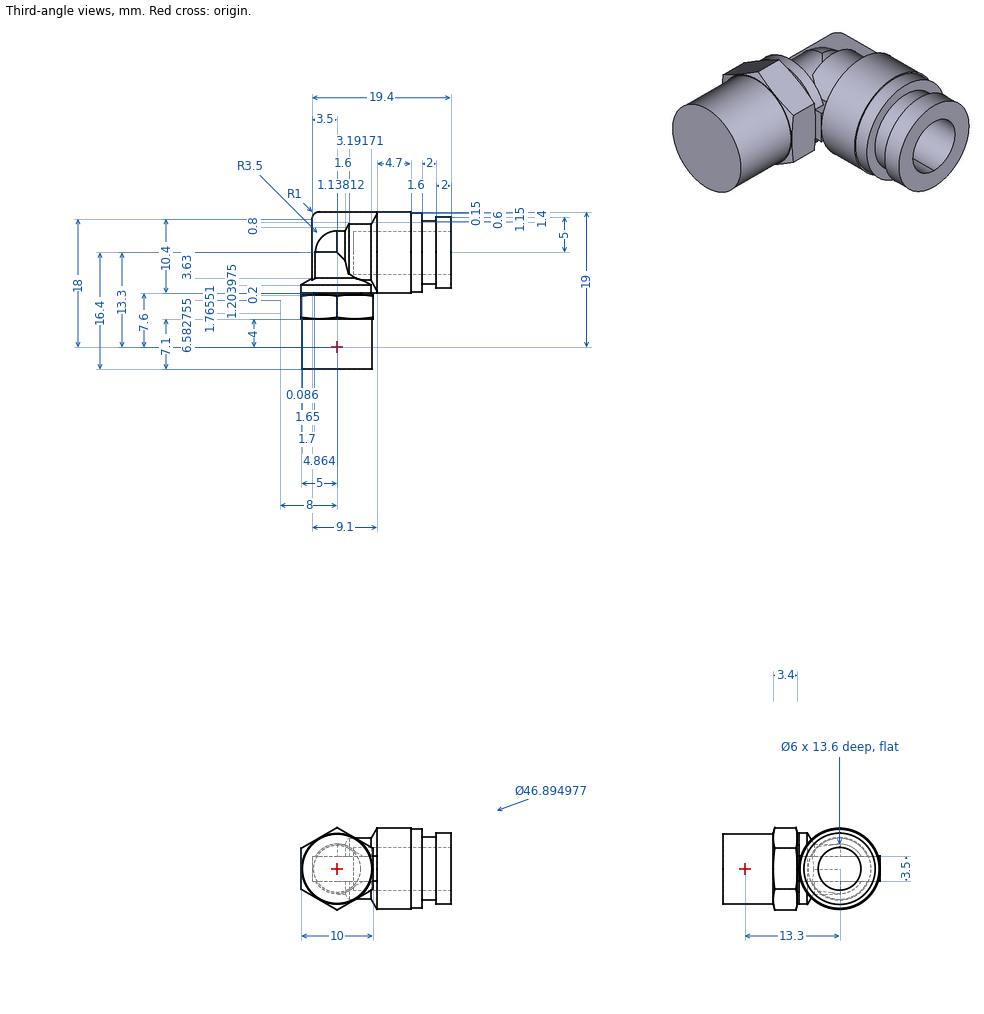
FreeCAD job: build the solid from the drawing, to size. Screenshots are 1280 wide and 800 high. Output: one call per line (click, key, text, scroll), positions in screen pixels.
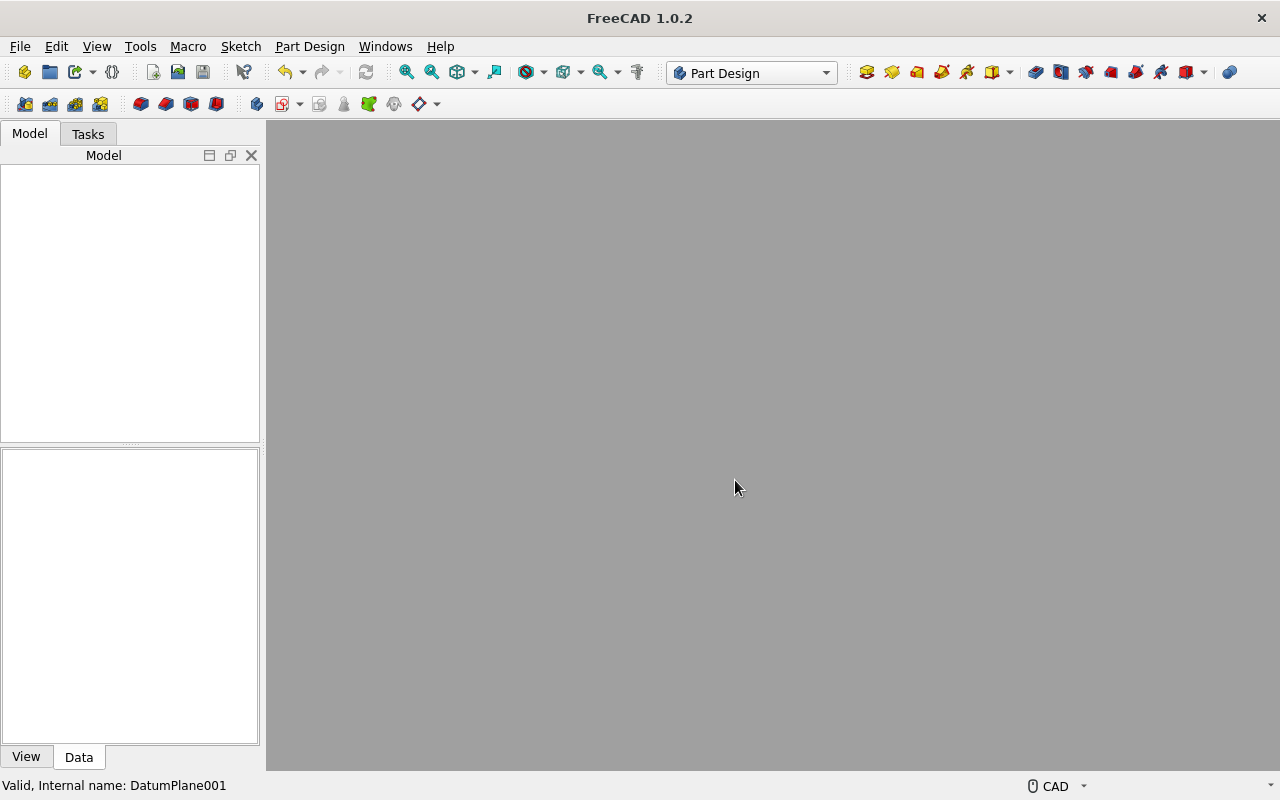
key(ctrl+n)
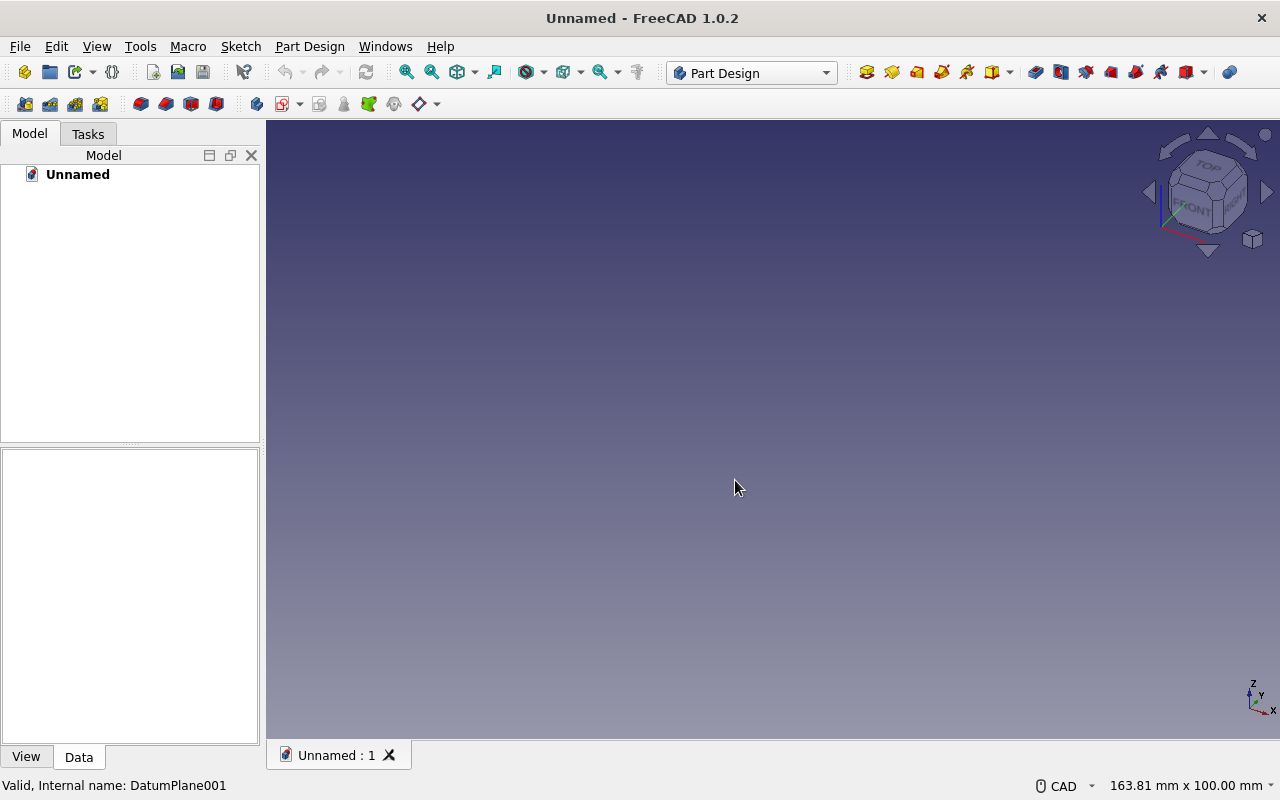
click(282, 104)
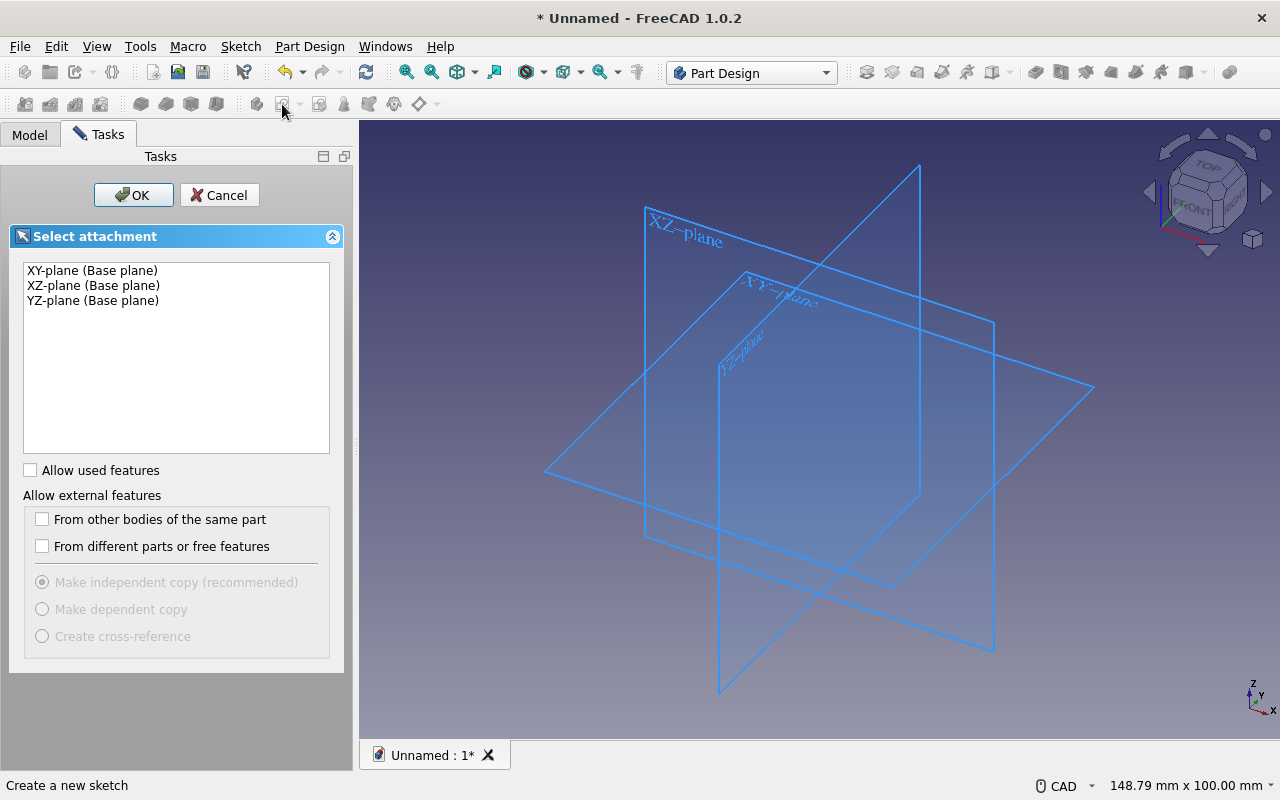
click(84, 270)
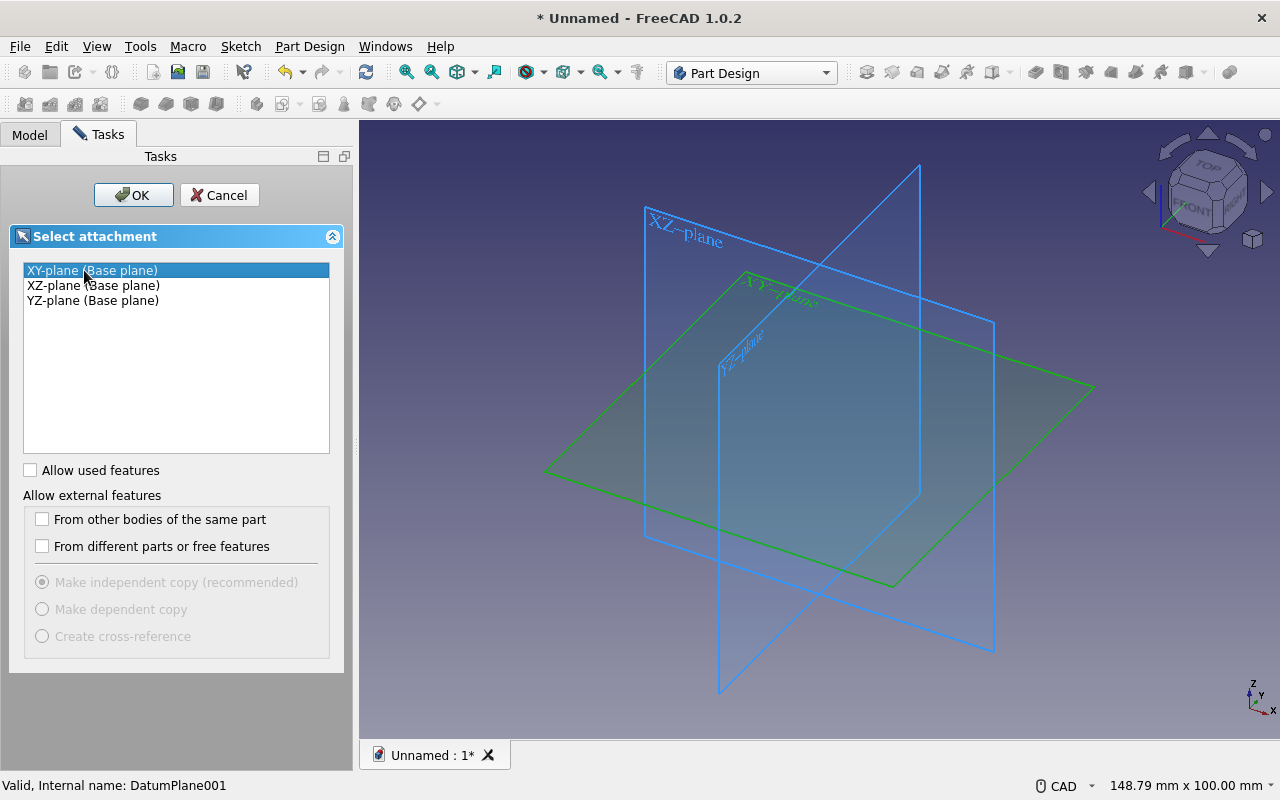
click(134, 195)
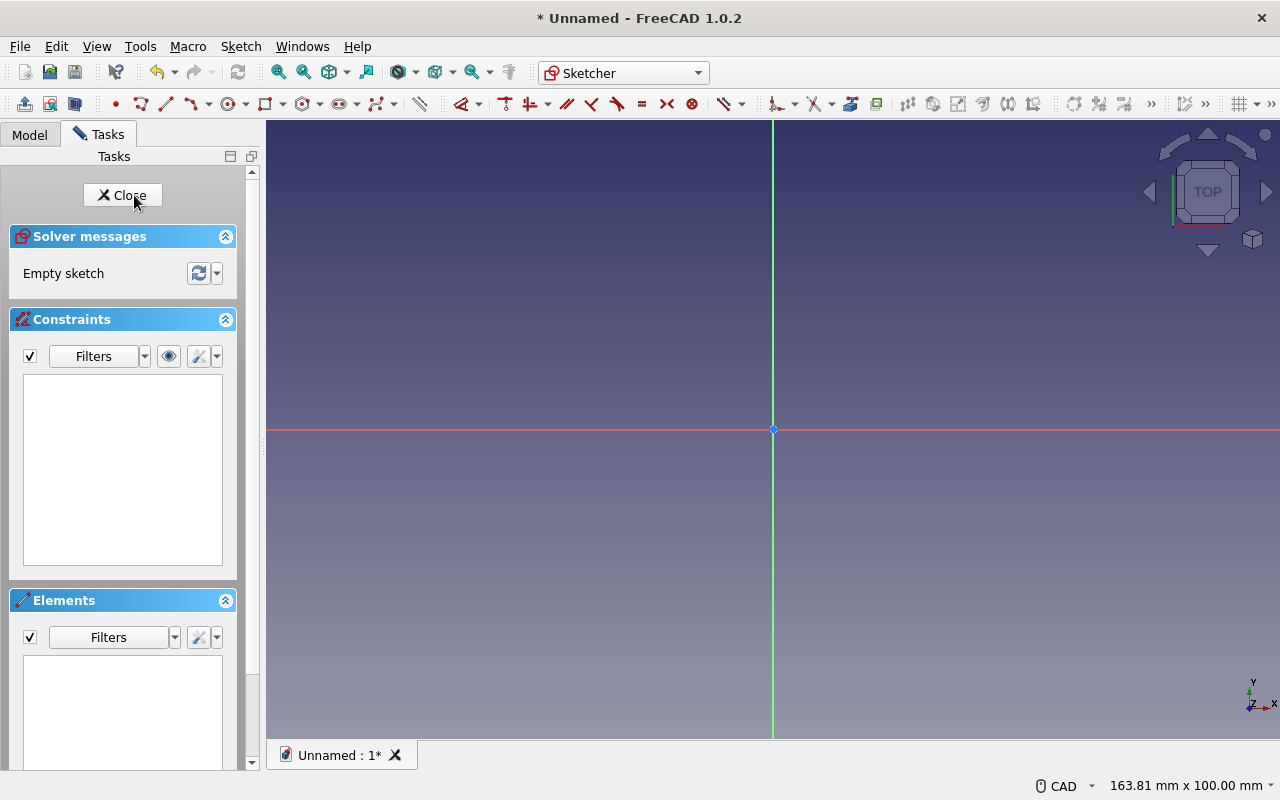
scroll(763, 388, up, 7)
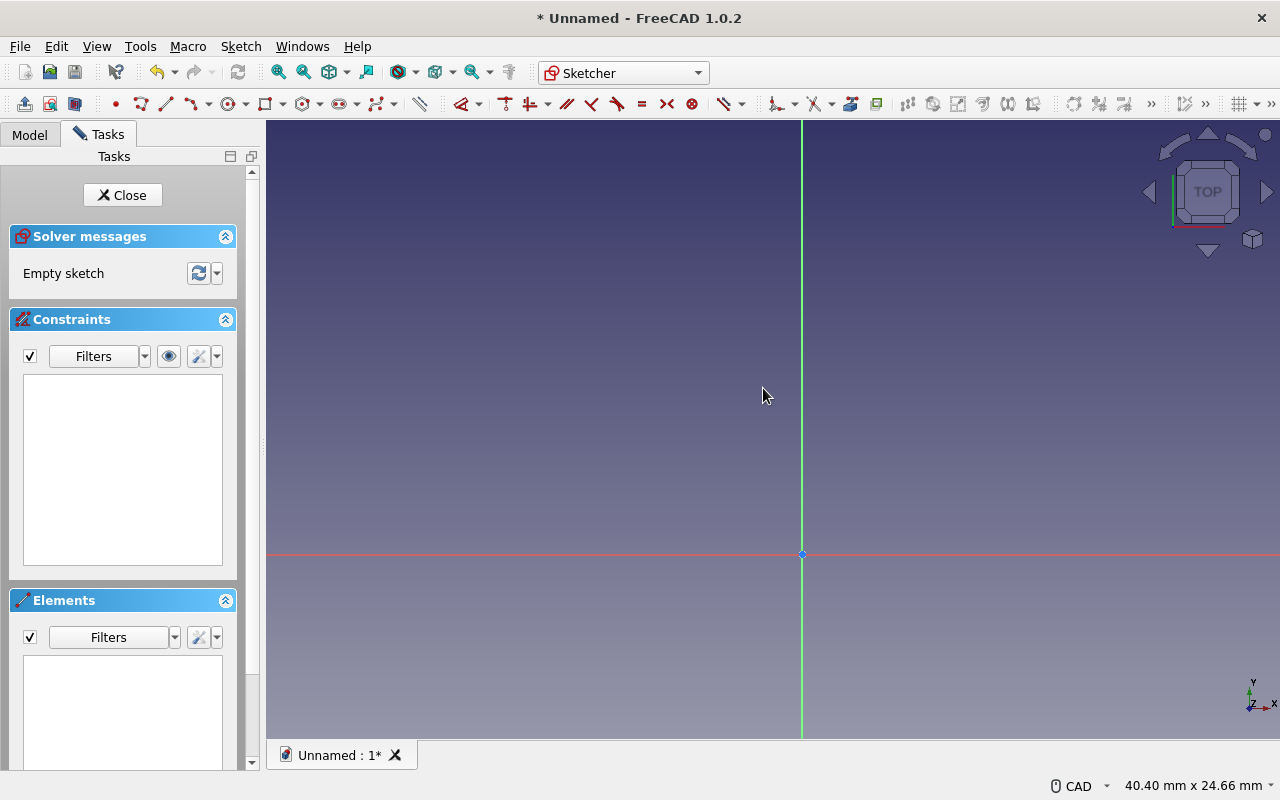
key(g)
key(m)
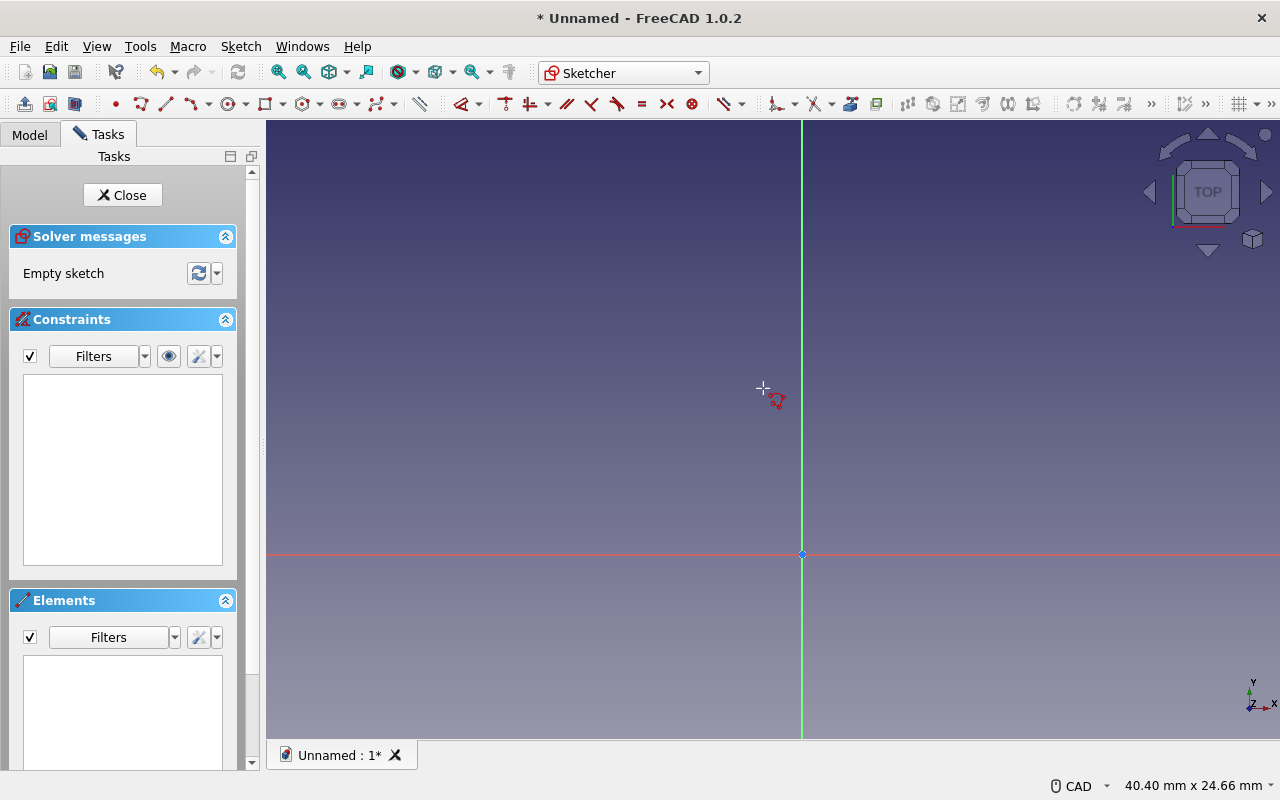
click(802, 633)
click(793, 221)
click(714, 221)
click(714, 312)
click(677, 334)
click(677, 364)
click(719, 364)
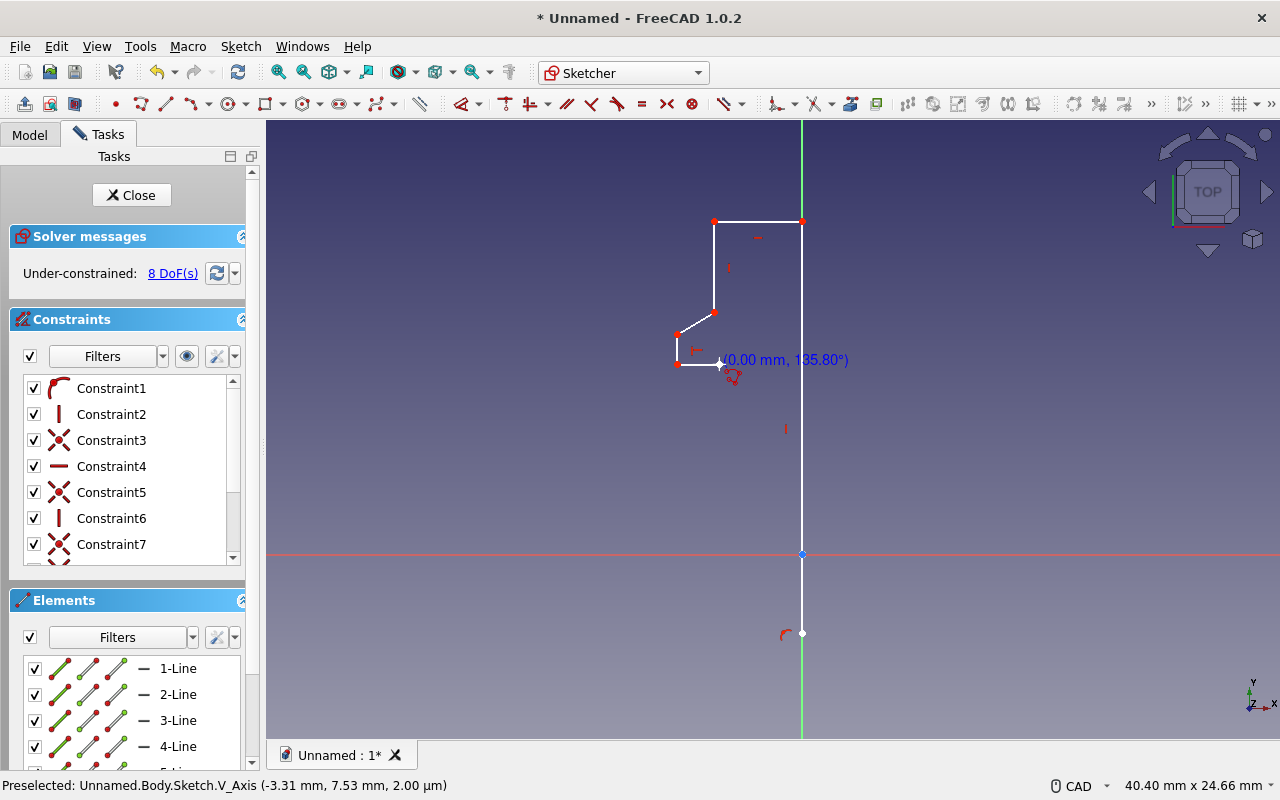
scroll(719, 369, up, 6)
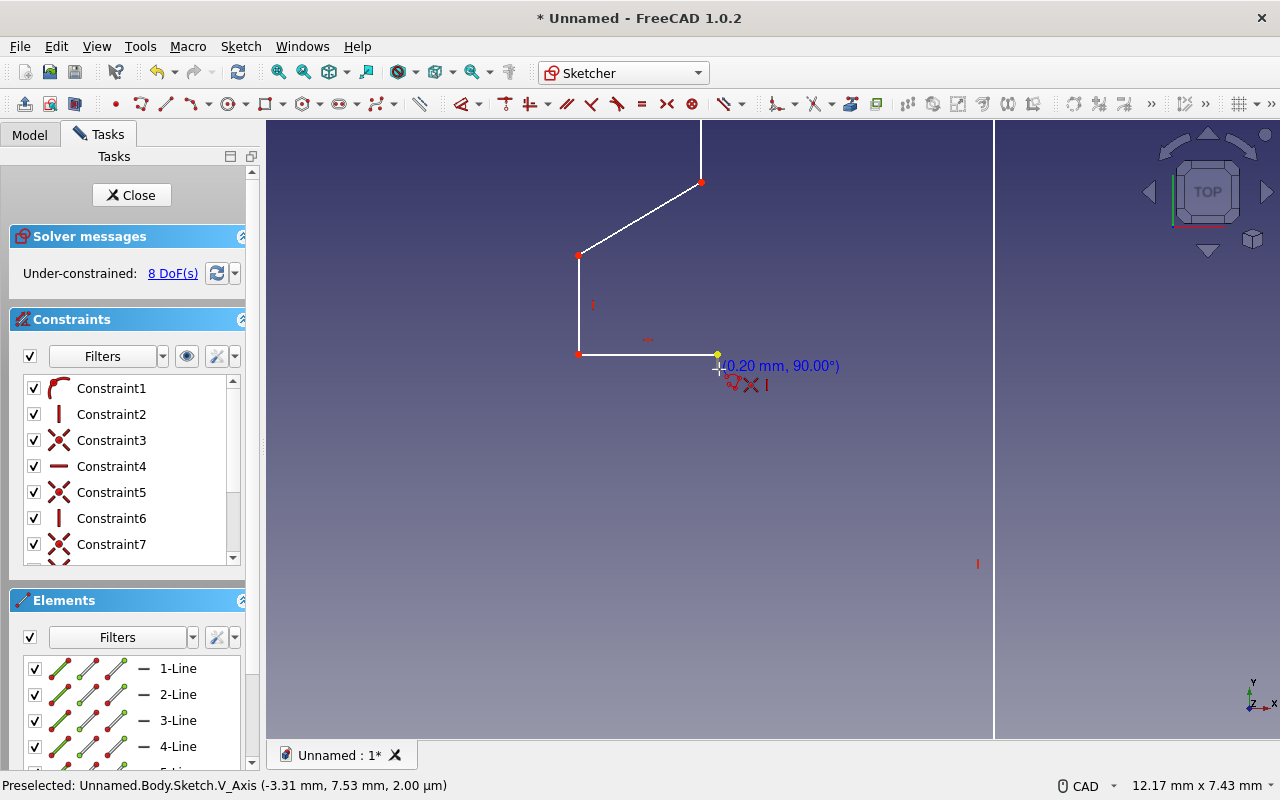
click(718, 369)
click(581, 369)
click(327, 437)
click(327, 584)
click(581, 652)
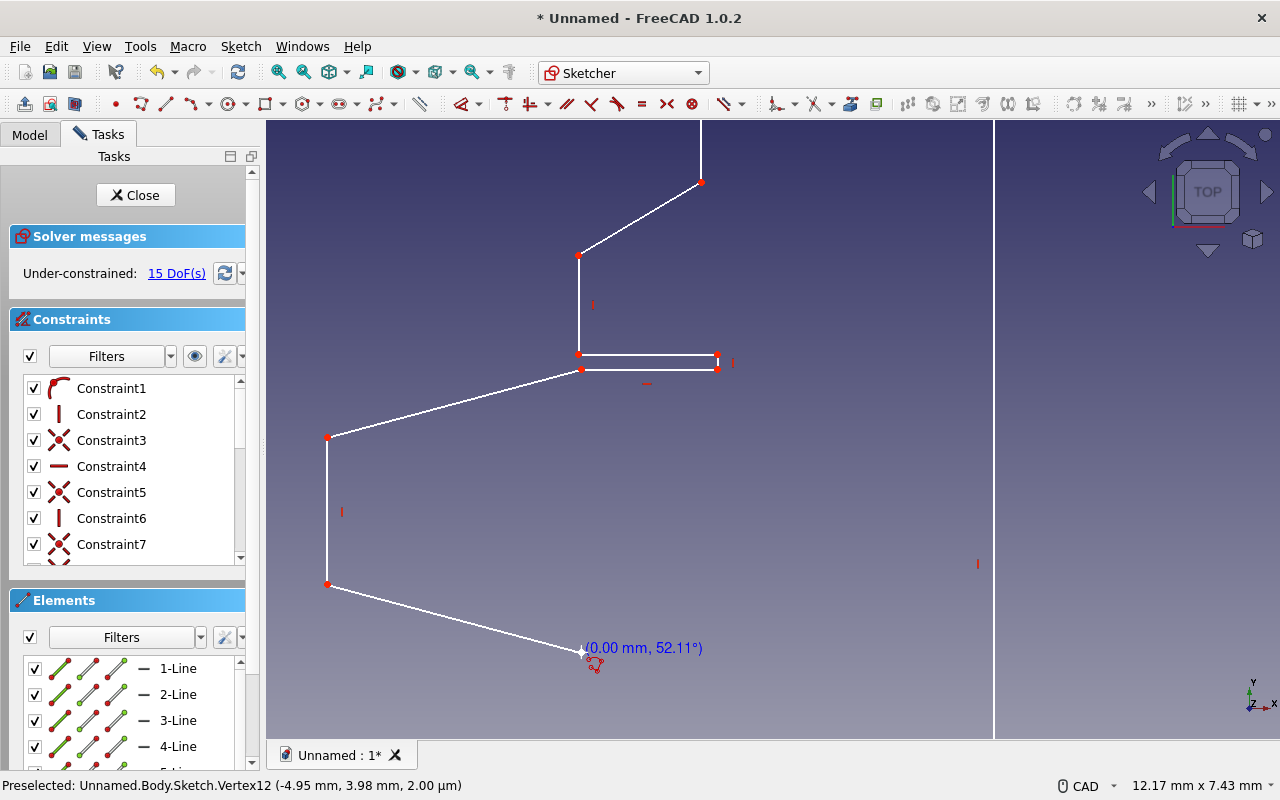
scroll(588, 652, up, 4)